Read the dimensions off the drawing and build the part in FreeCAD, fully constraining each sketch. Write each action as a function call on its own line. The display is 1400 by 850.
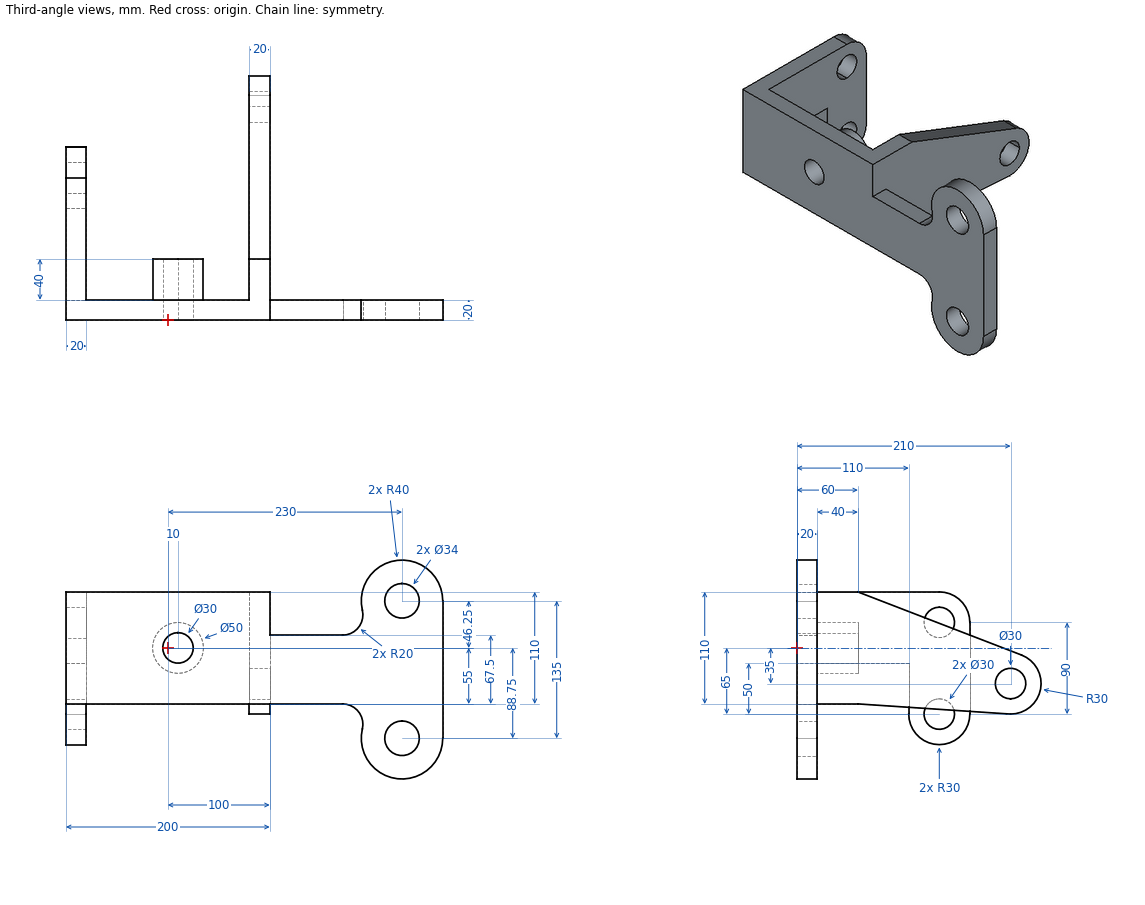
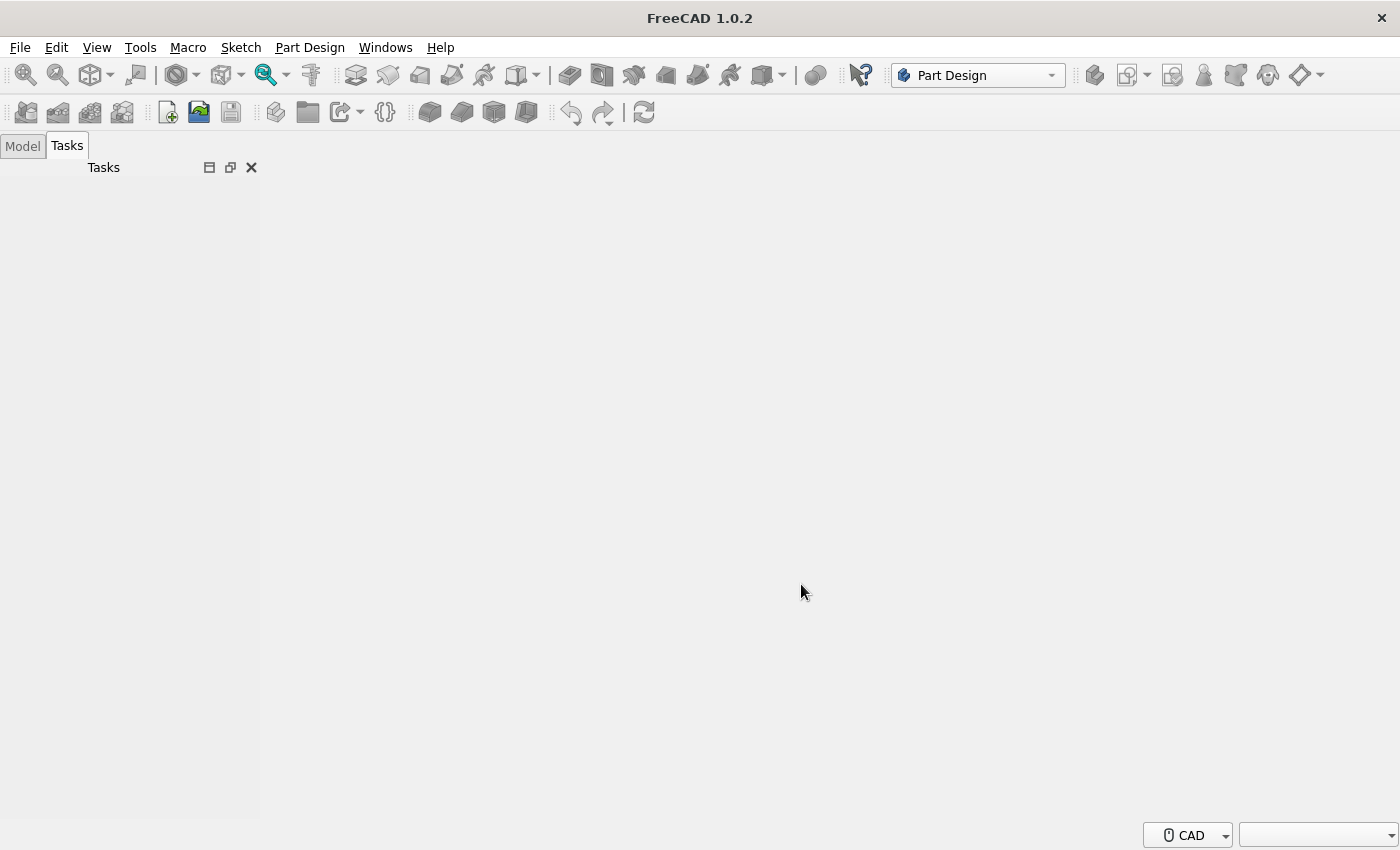
click(168, 112)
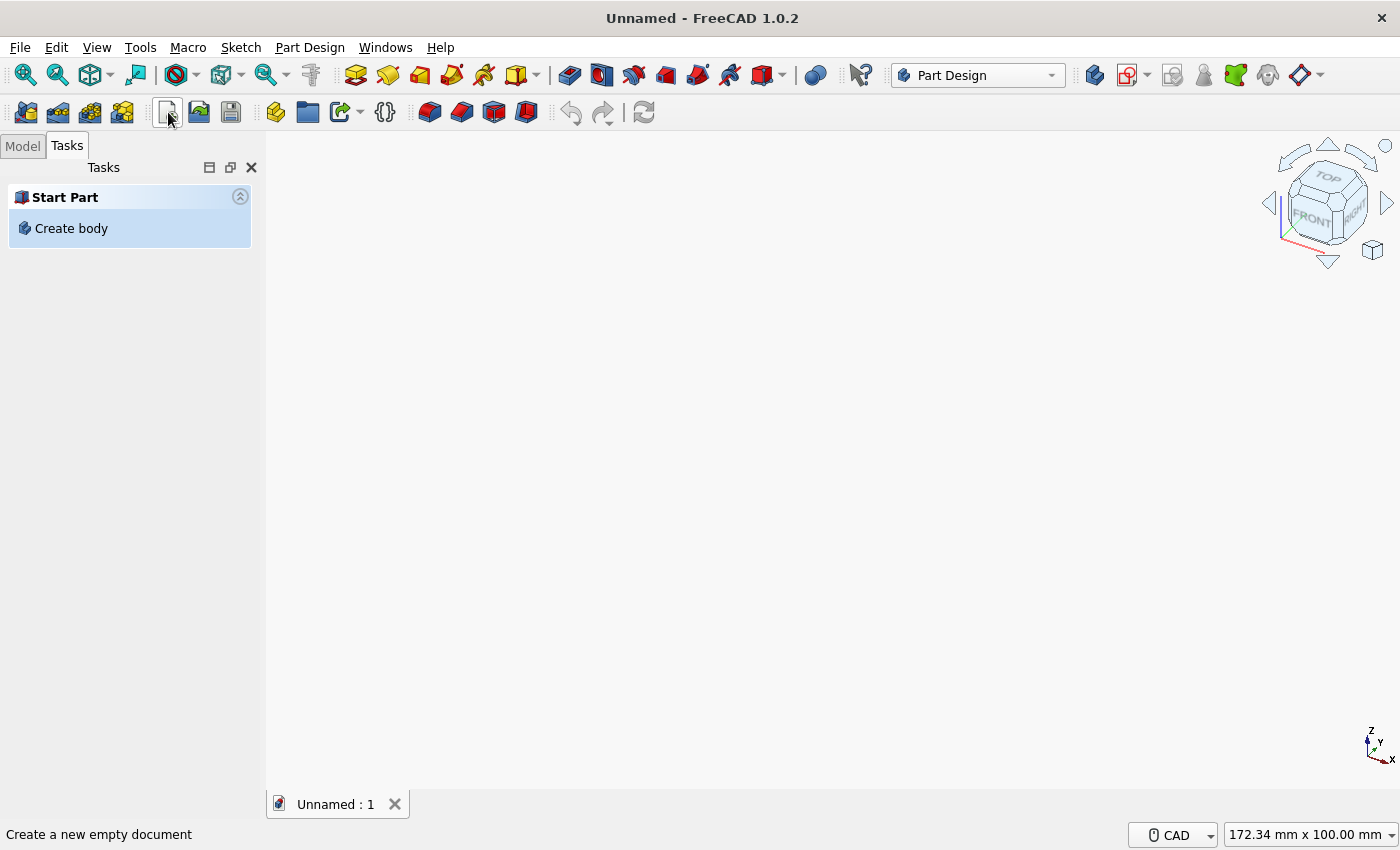
click(1128, 76)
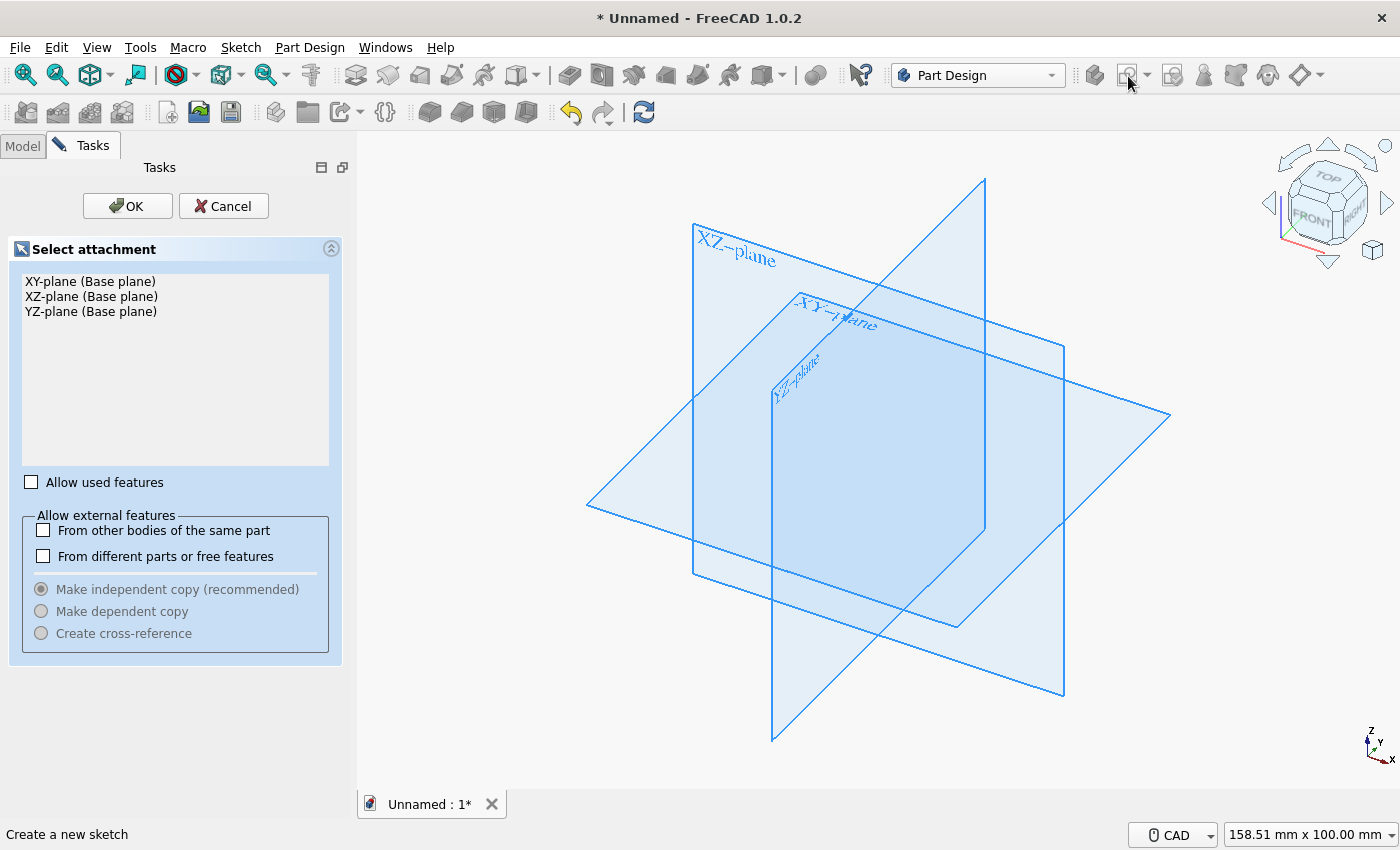
click(82, 296)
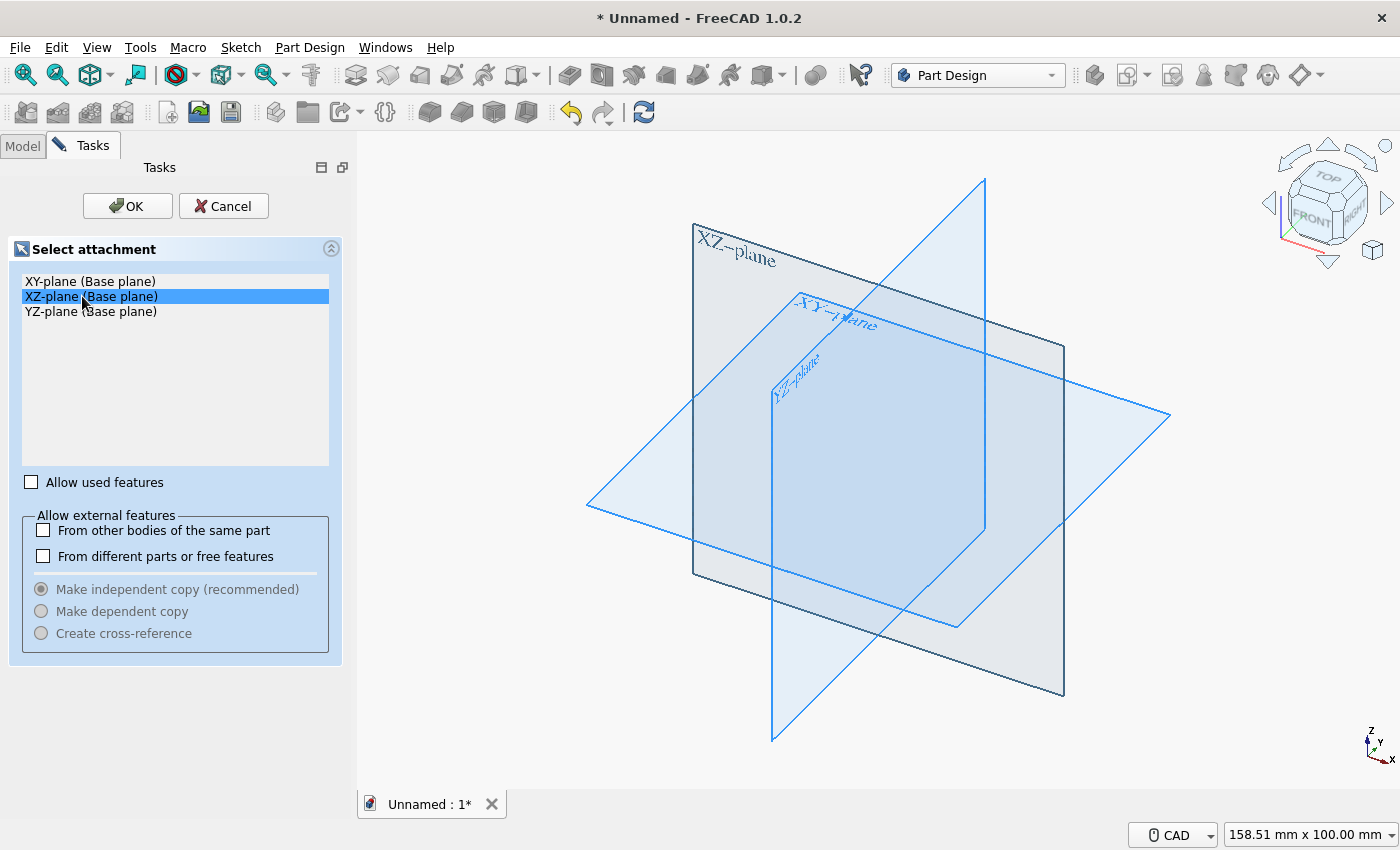
click(128, 206)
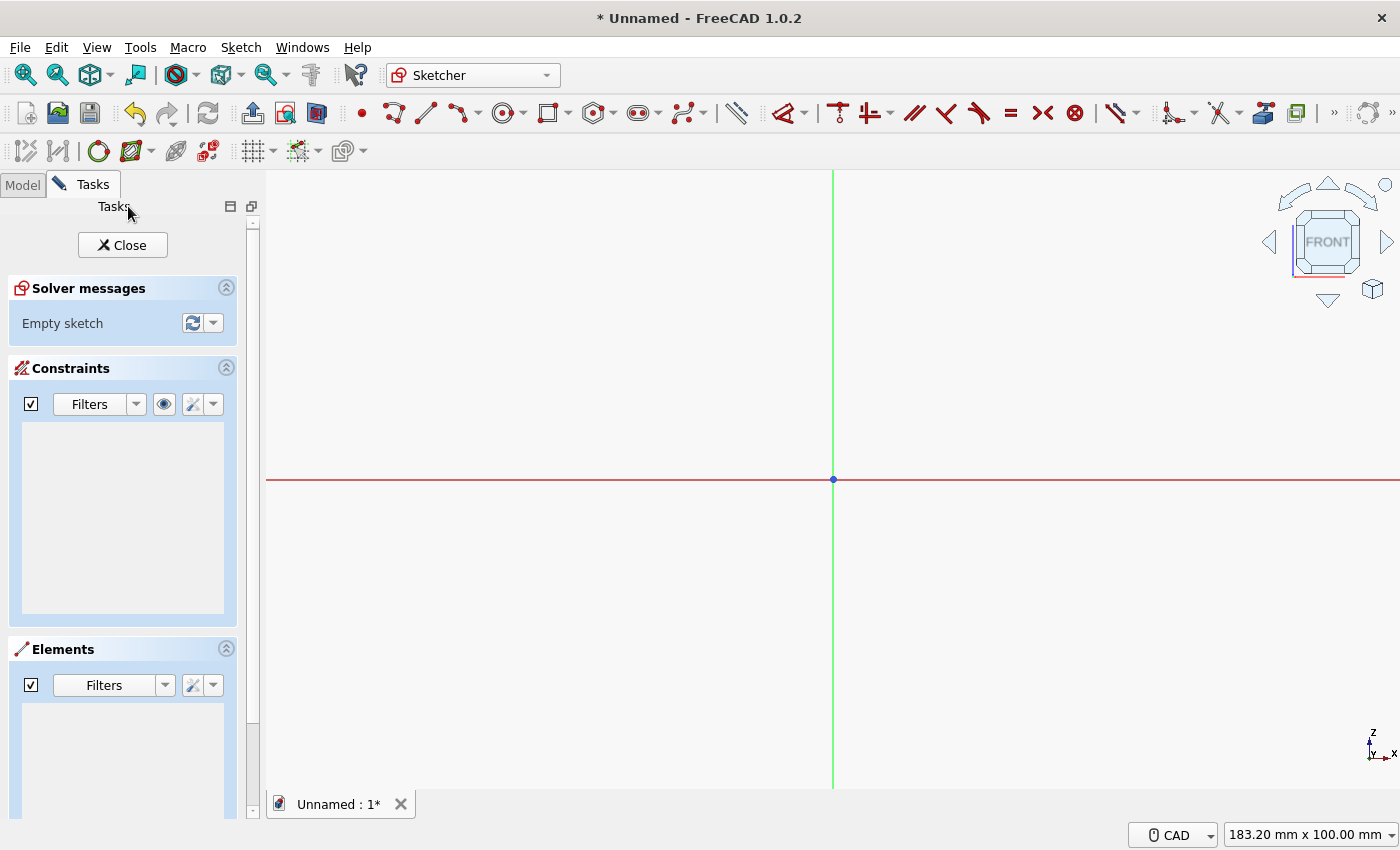
scroll(681, 479, down, 3)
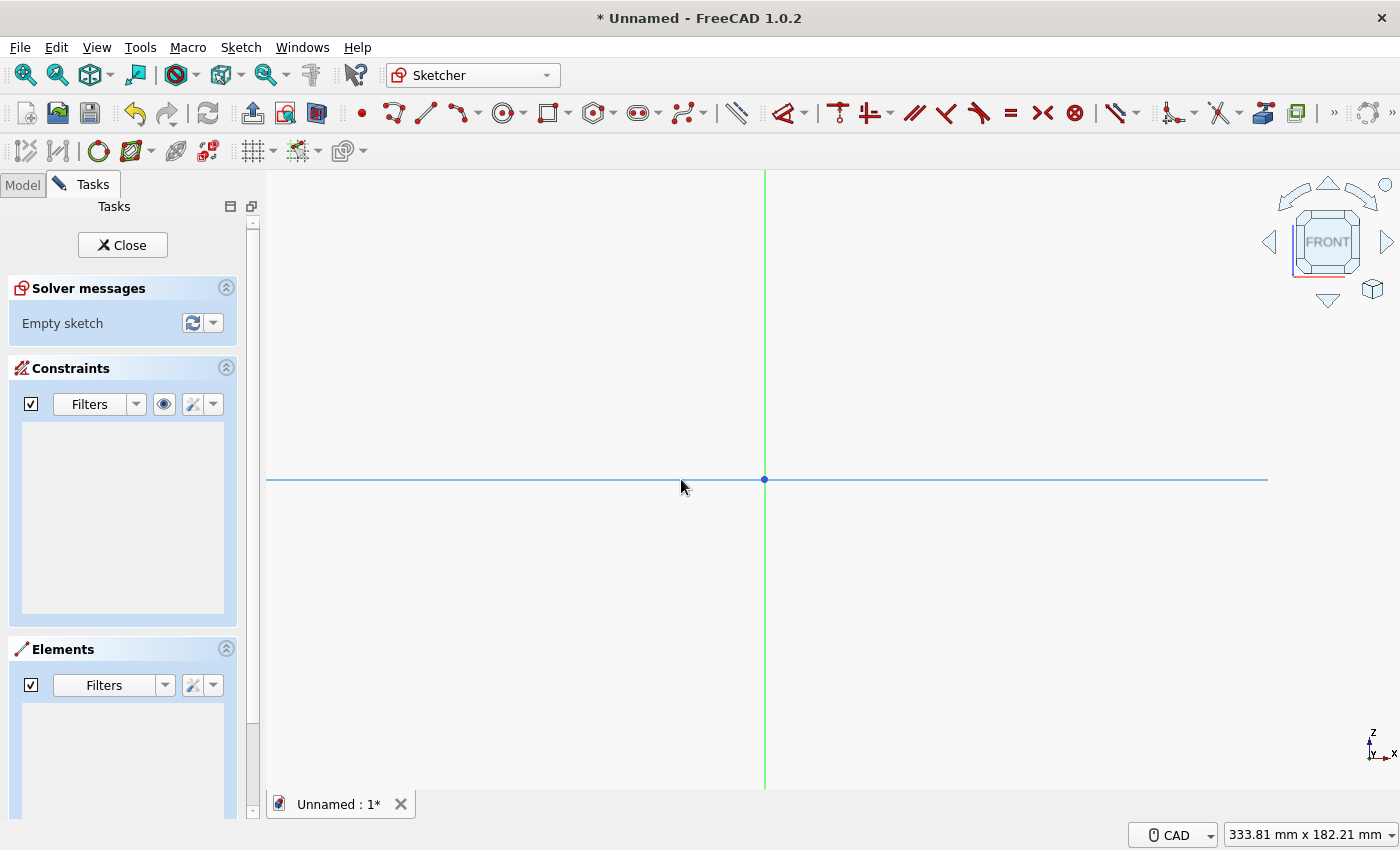
key(g)
key(v)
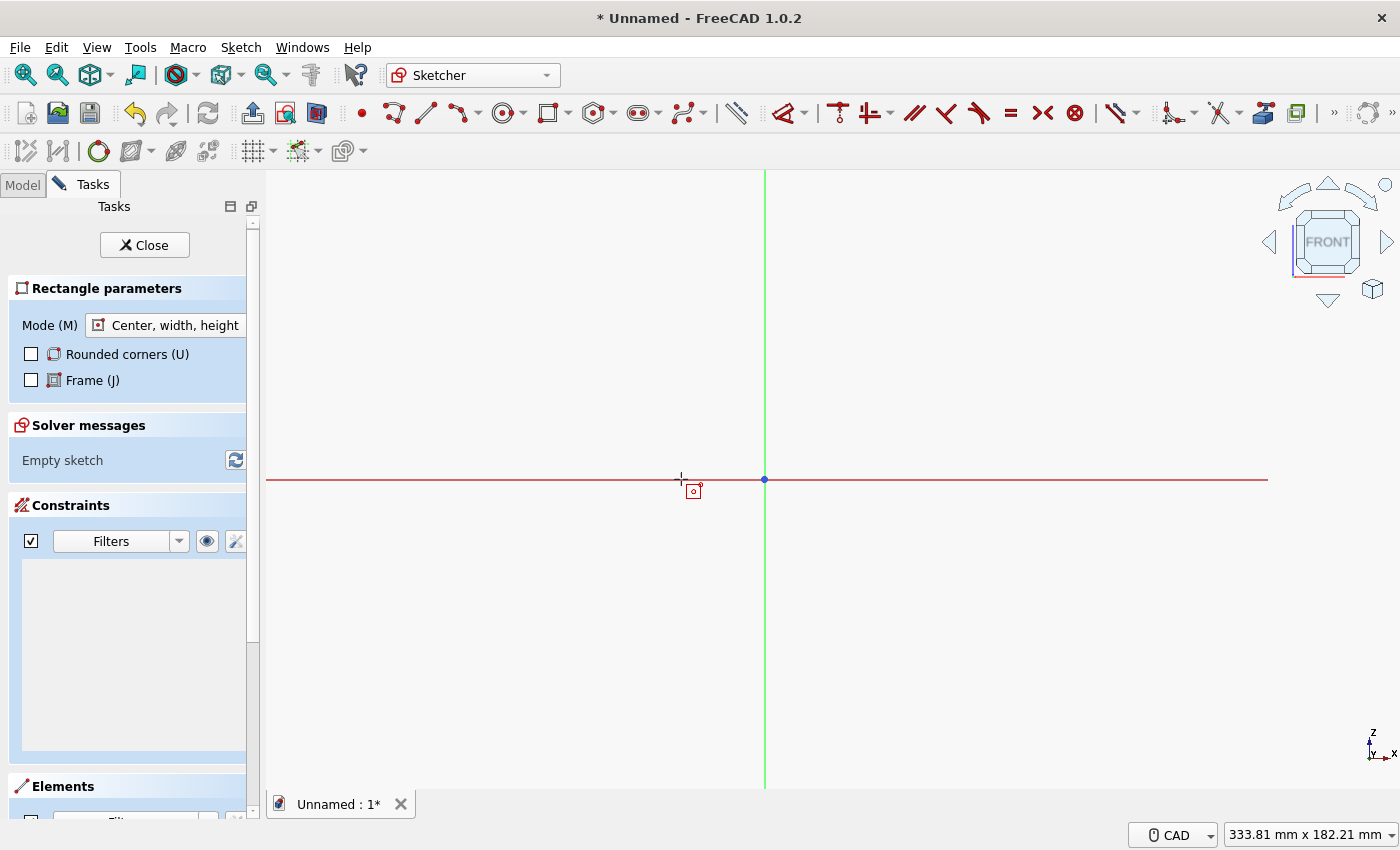
click(765, 480)
click(1104, 293)
key(Escape)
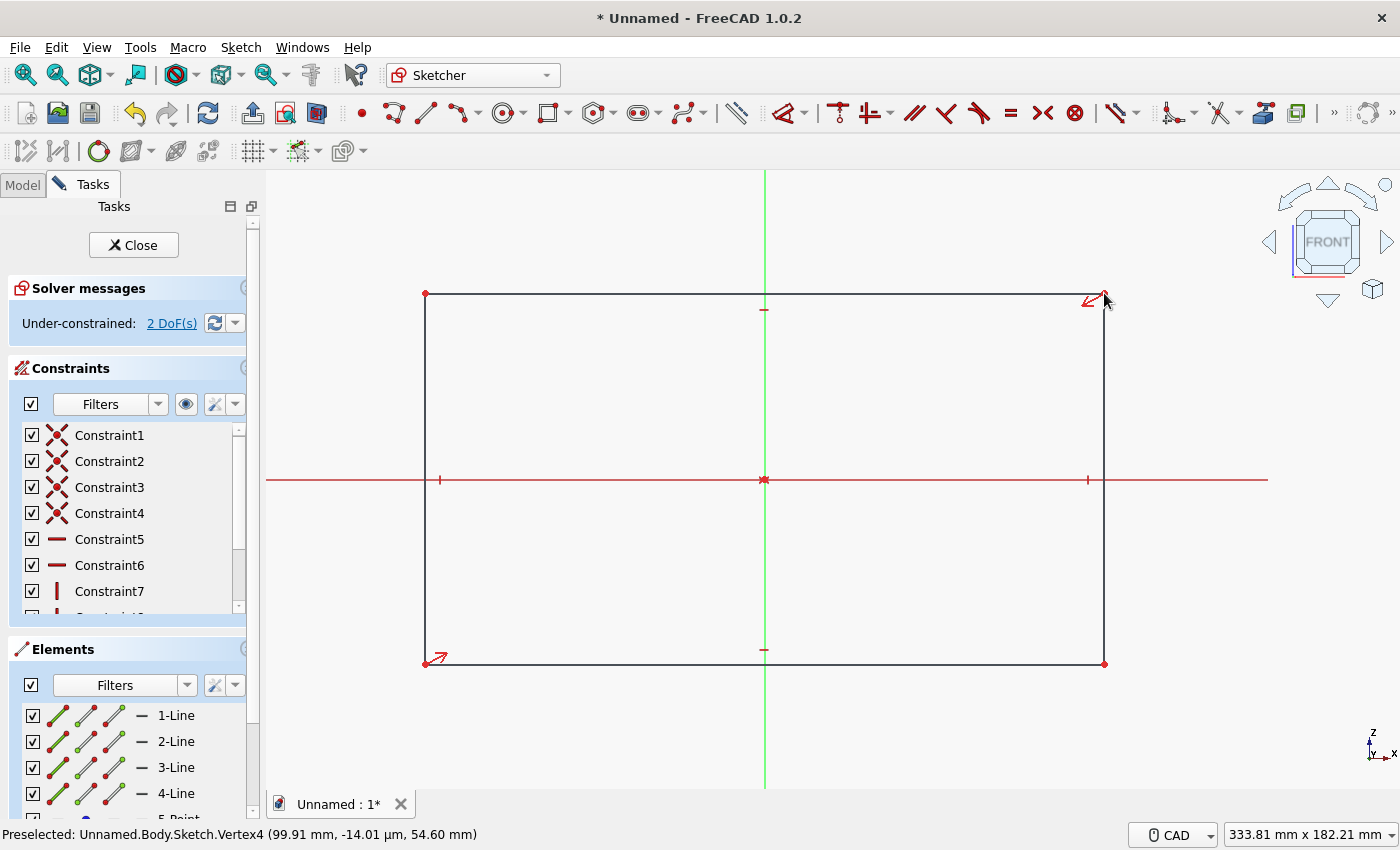
click(629, 665)